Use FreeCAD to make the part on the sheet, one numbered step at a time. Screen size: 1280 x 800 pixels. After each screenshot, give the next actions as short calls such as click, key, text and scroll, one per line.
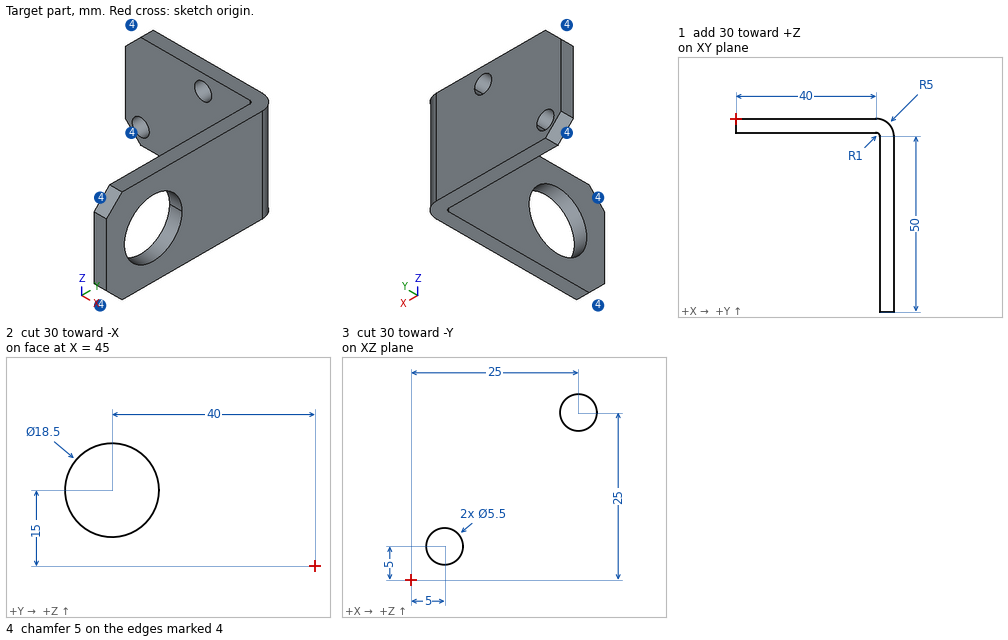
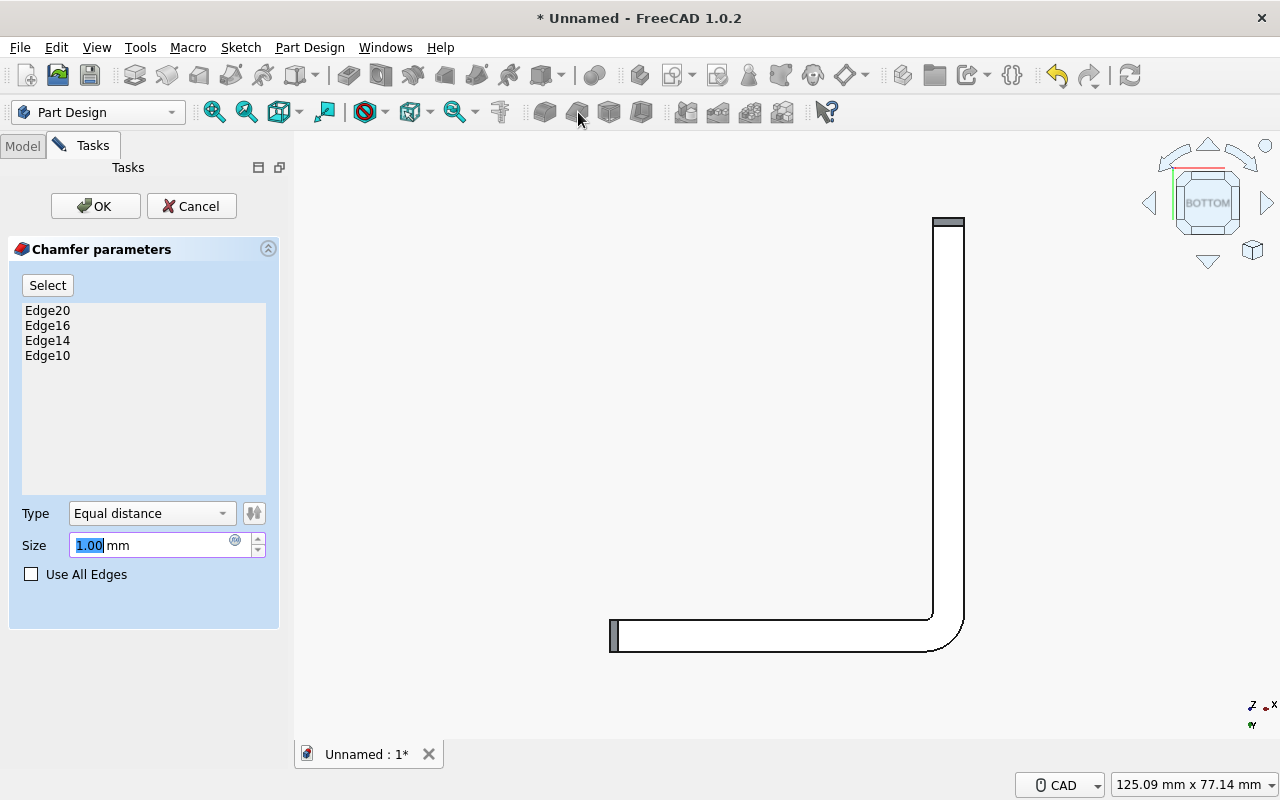
text(5)
key(Tab)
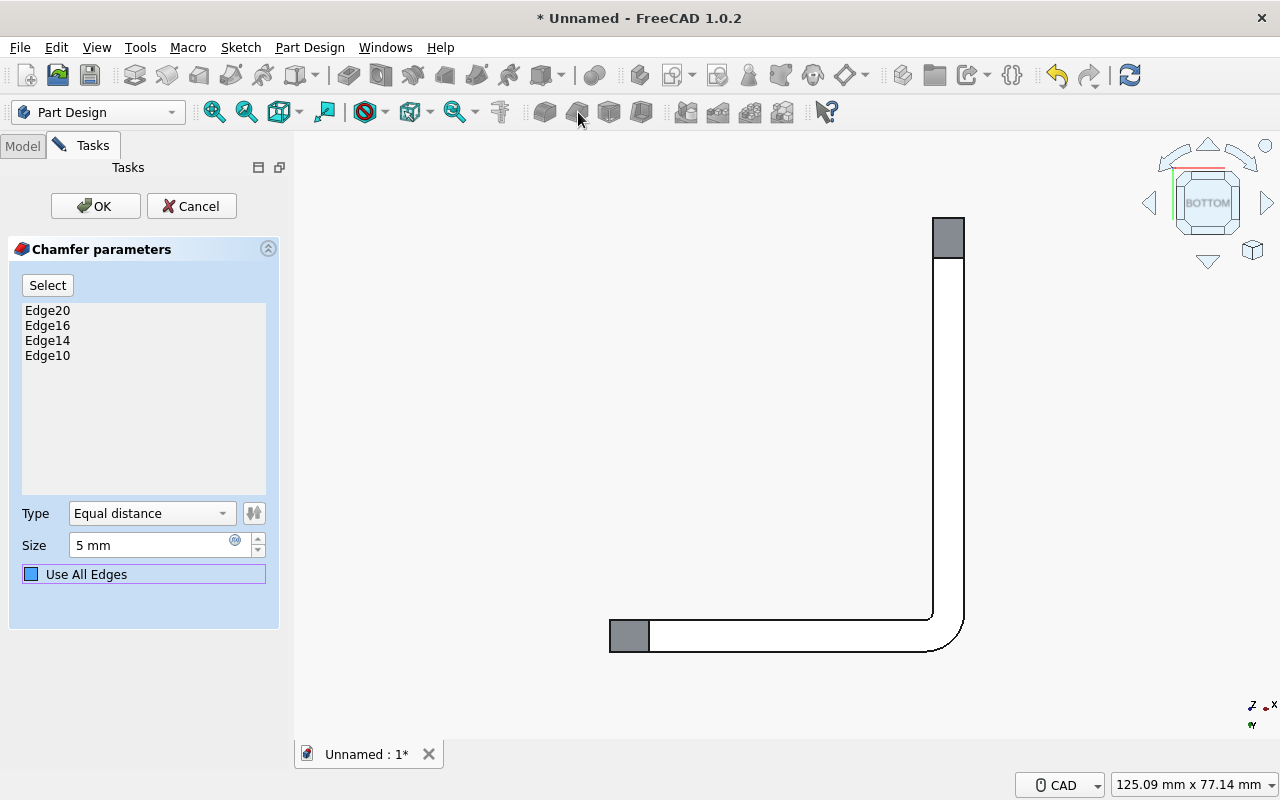
click(96, 206)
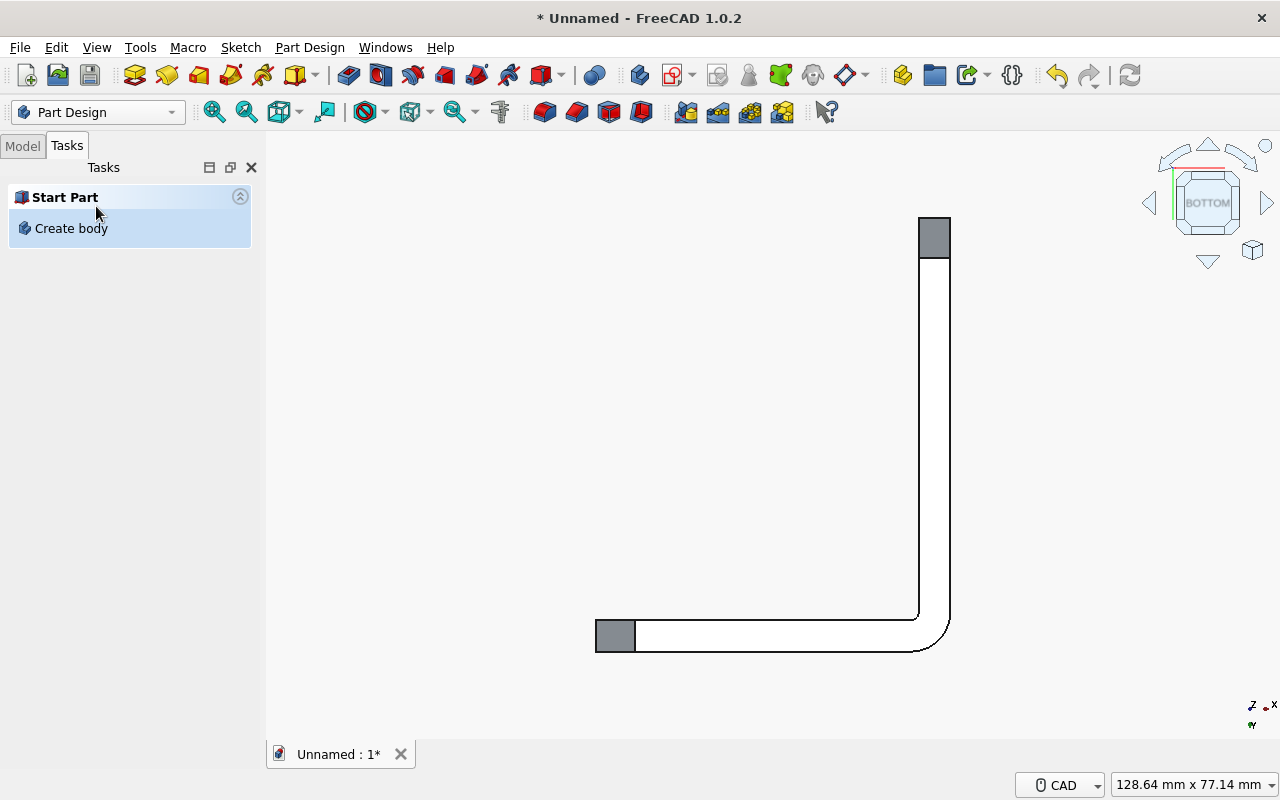
key(0)